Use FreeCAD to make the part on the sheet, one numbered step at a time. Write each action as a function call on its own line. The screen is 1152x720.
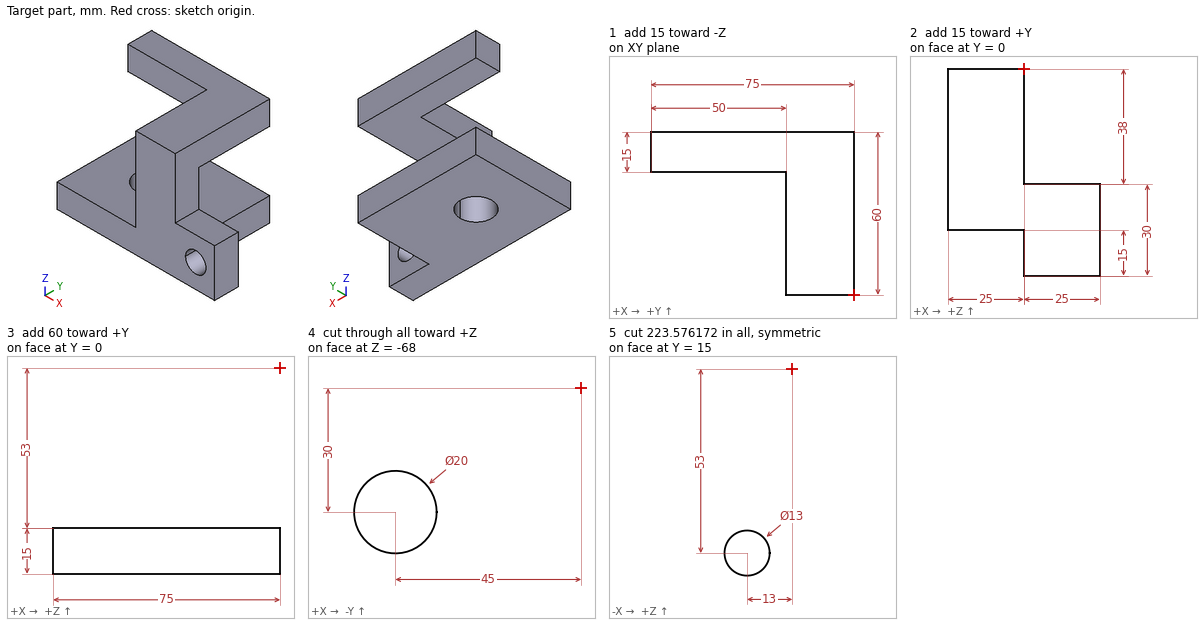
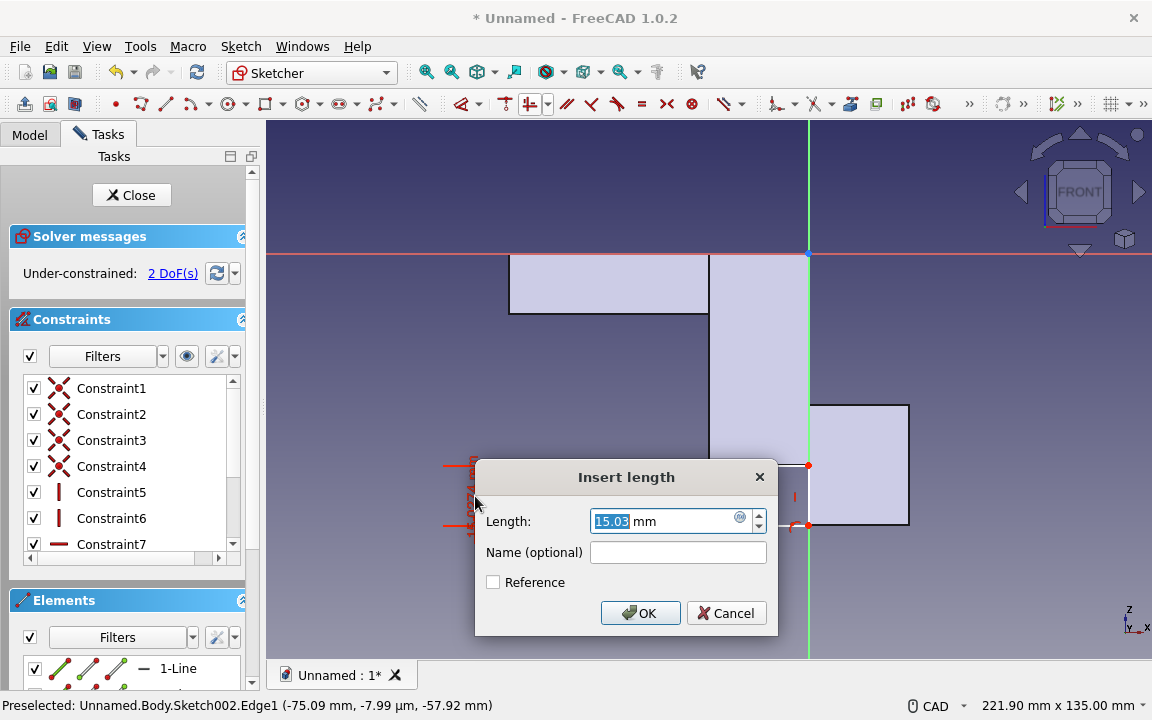
text(15)
key(Return)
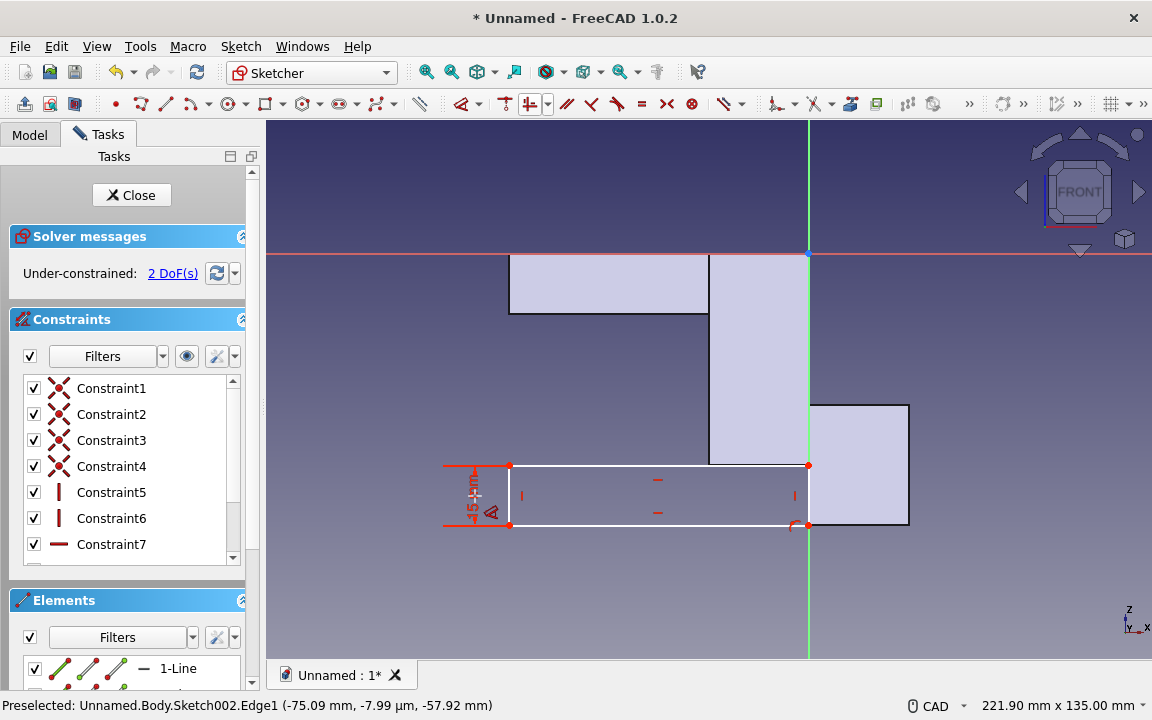
click(599, 526)
click(659, 560)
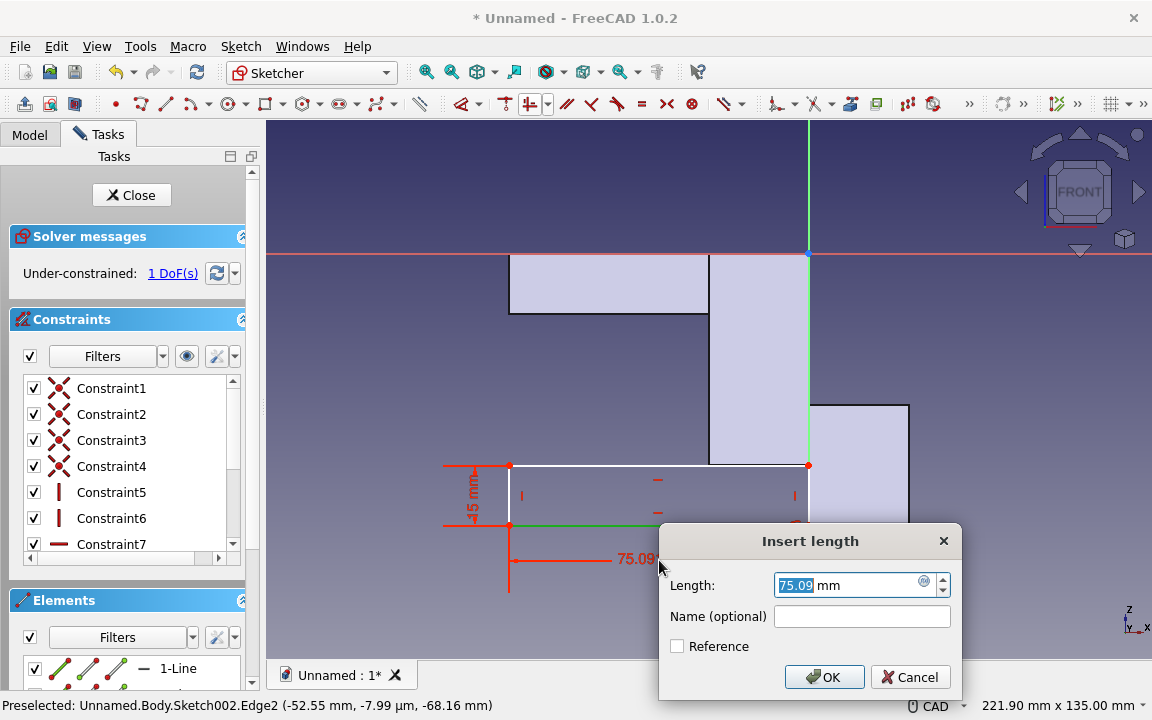
text(75)
key(Return)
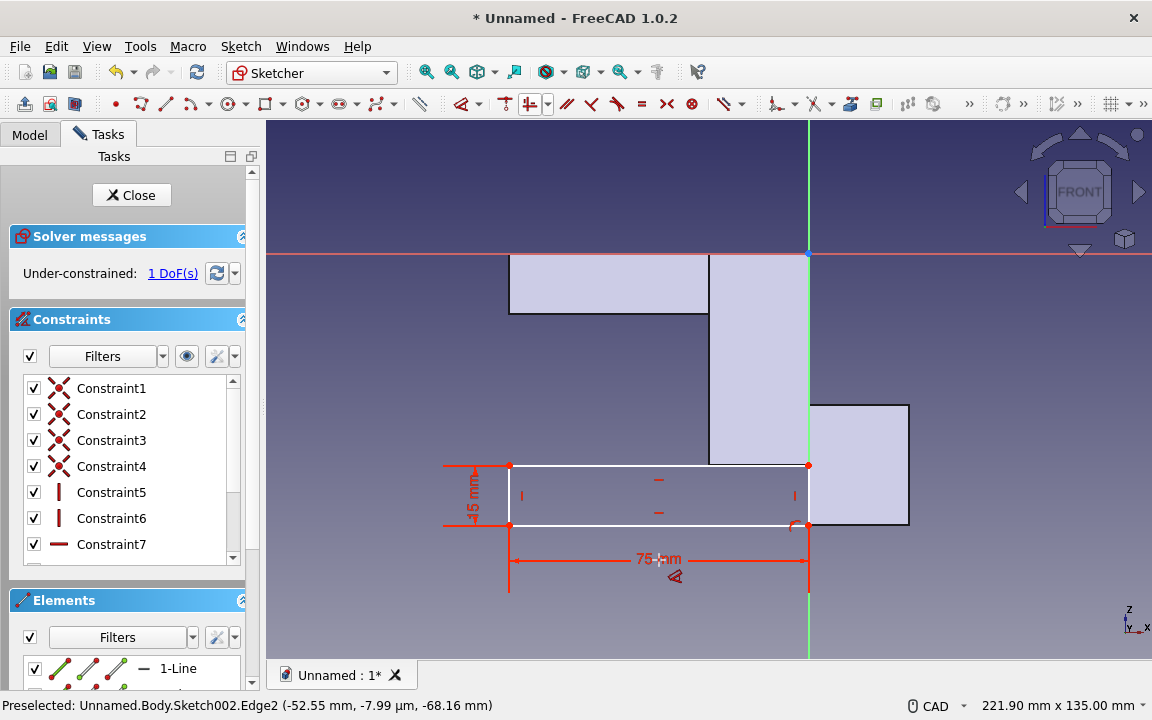
click(509, 466)
click(843, 360)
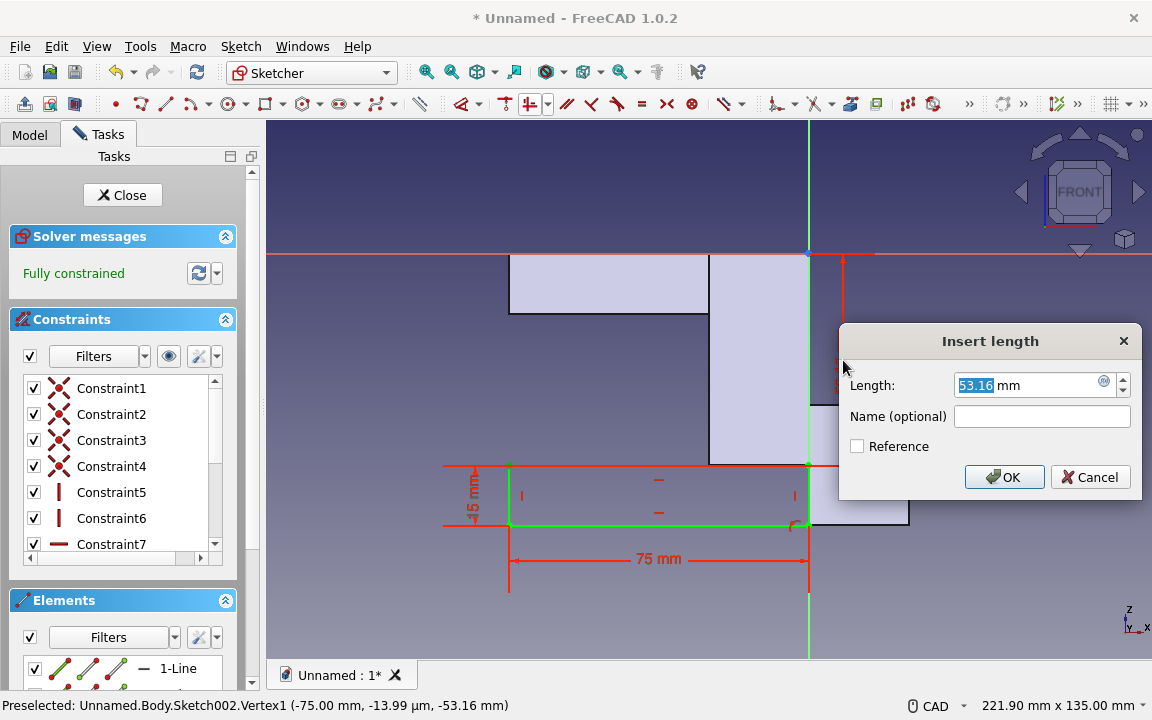
text(53)
key(Return)
key(Escape)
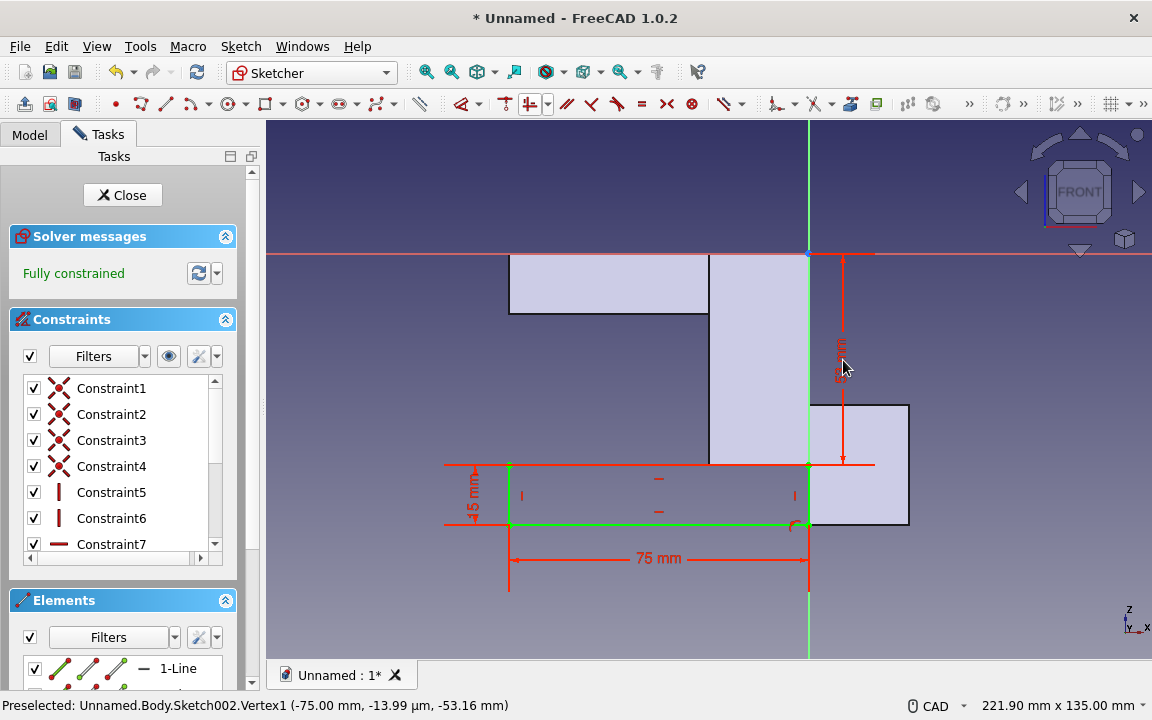
click(123, 195)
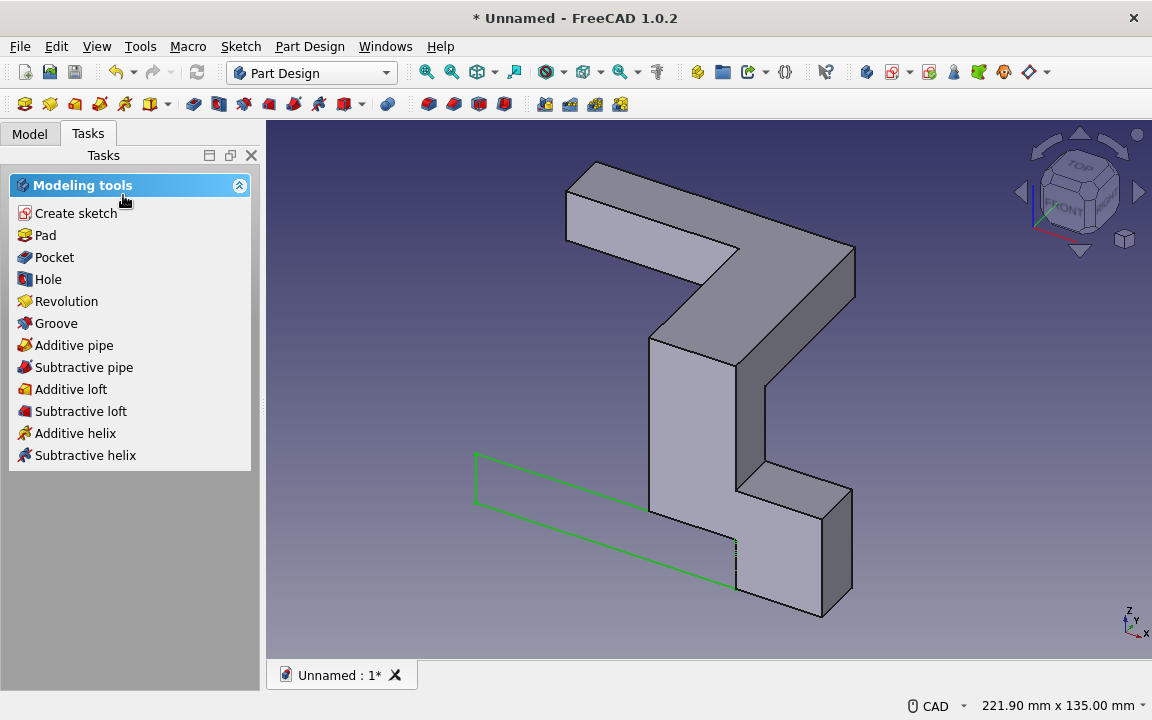
click(25, 104)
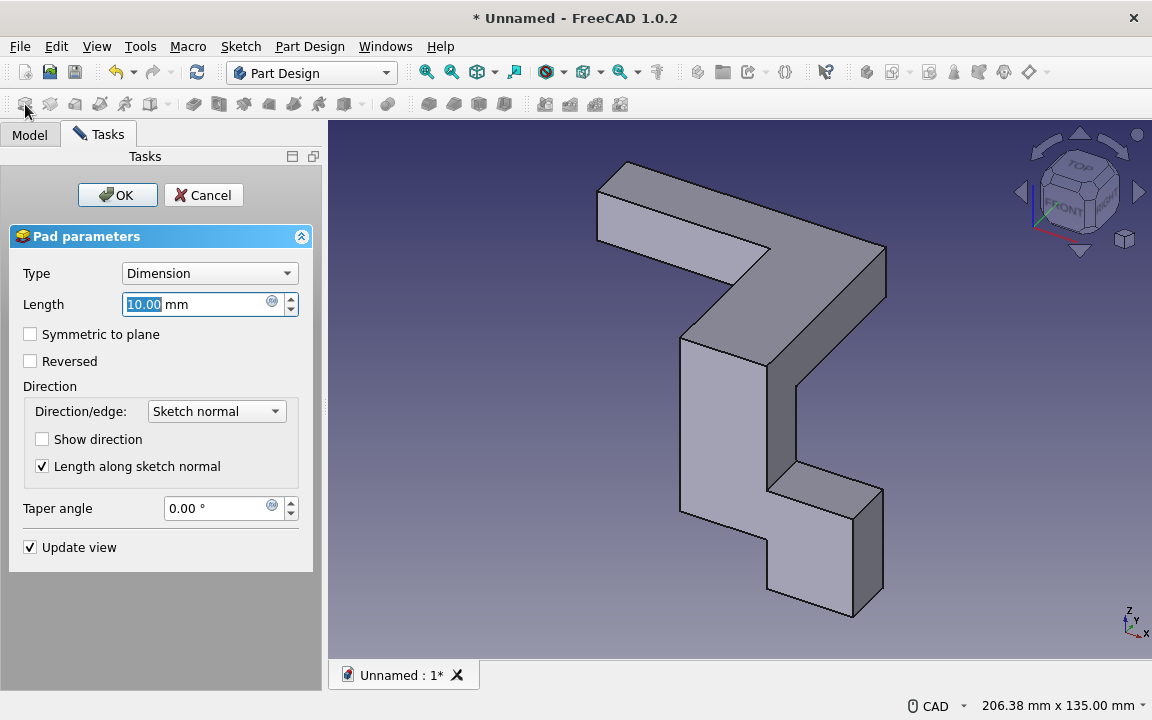
text(60)
key(Tab)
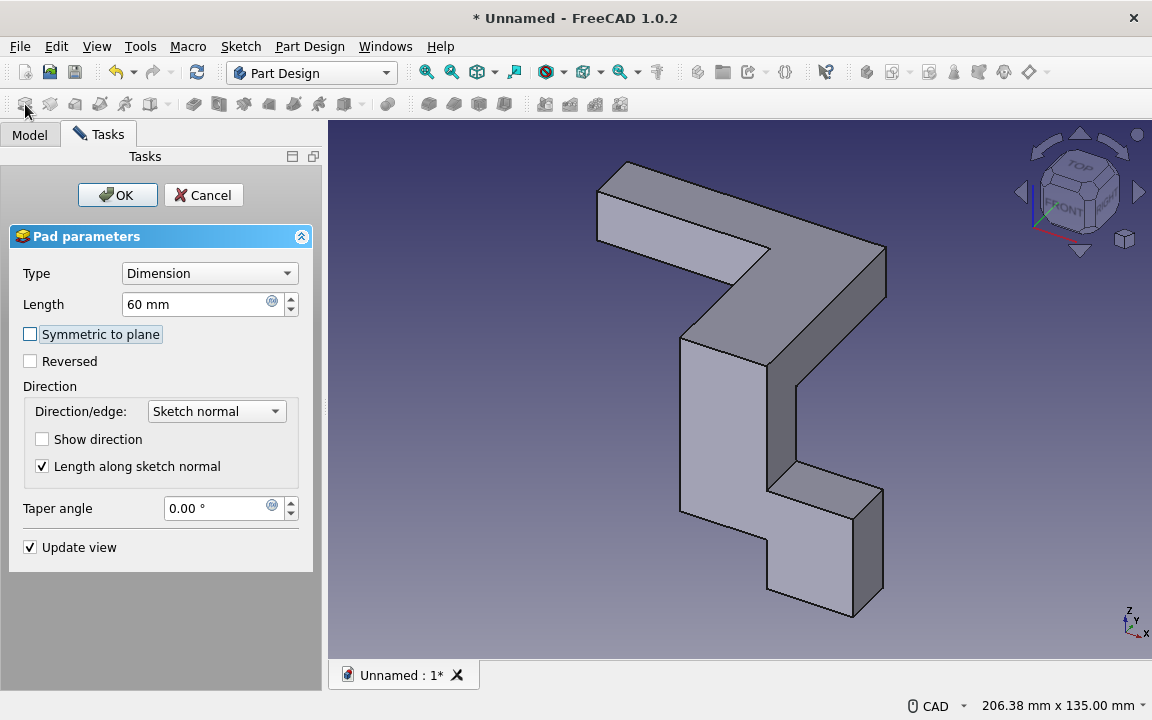
click(31, 361)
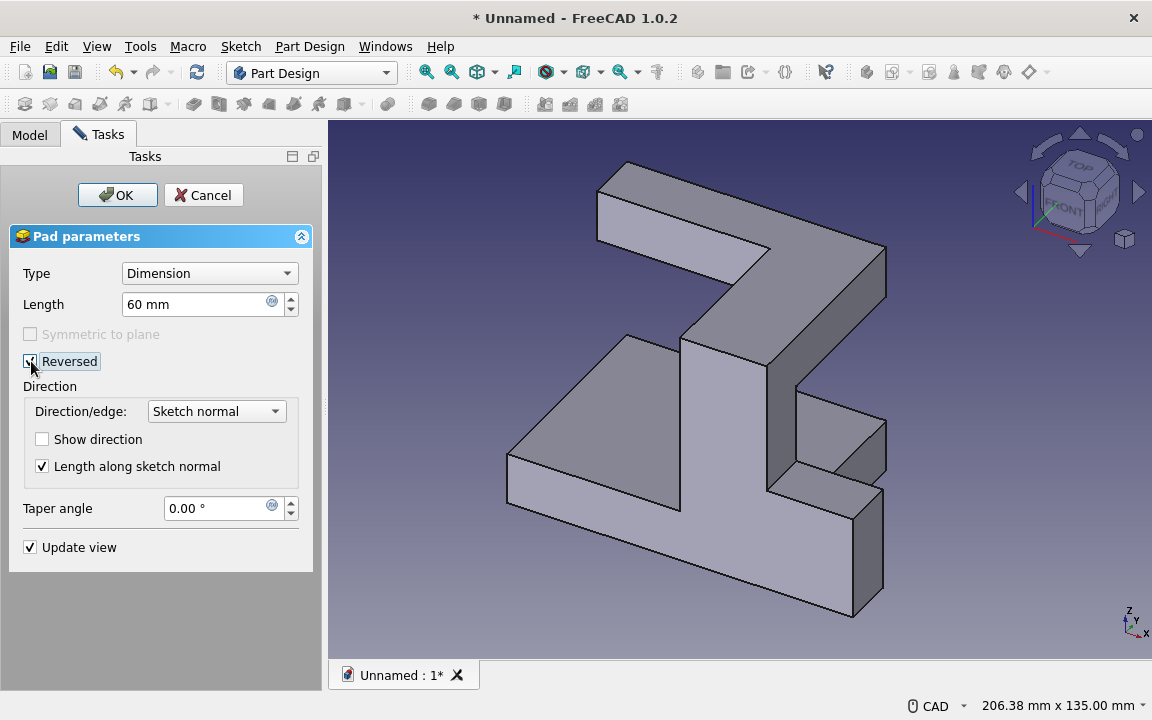
click(118, 195)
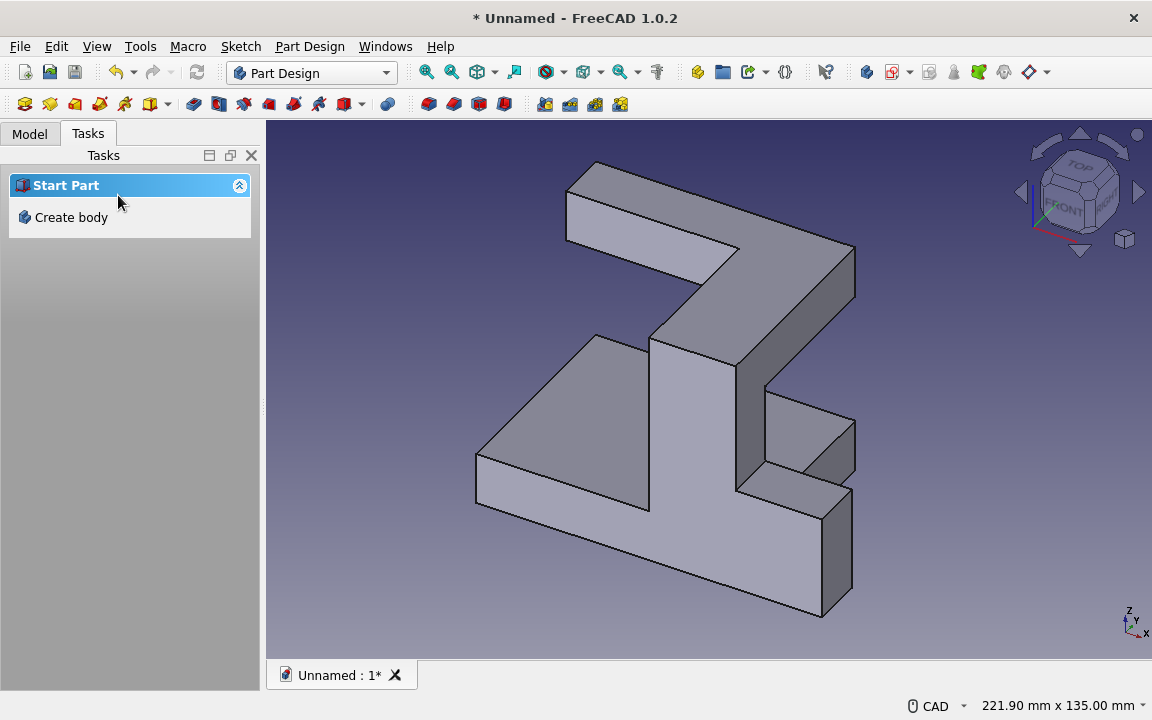
key(5)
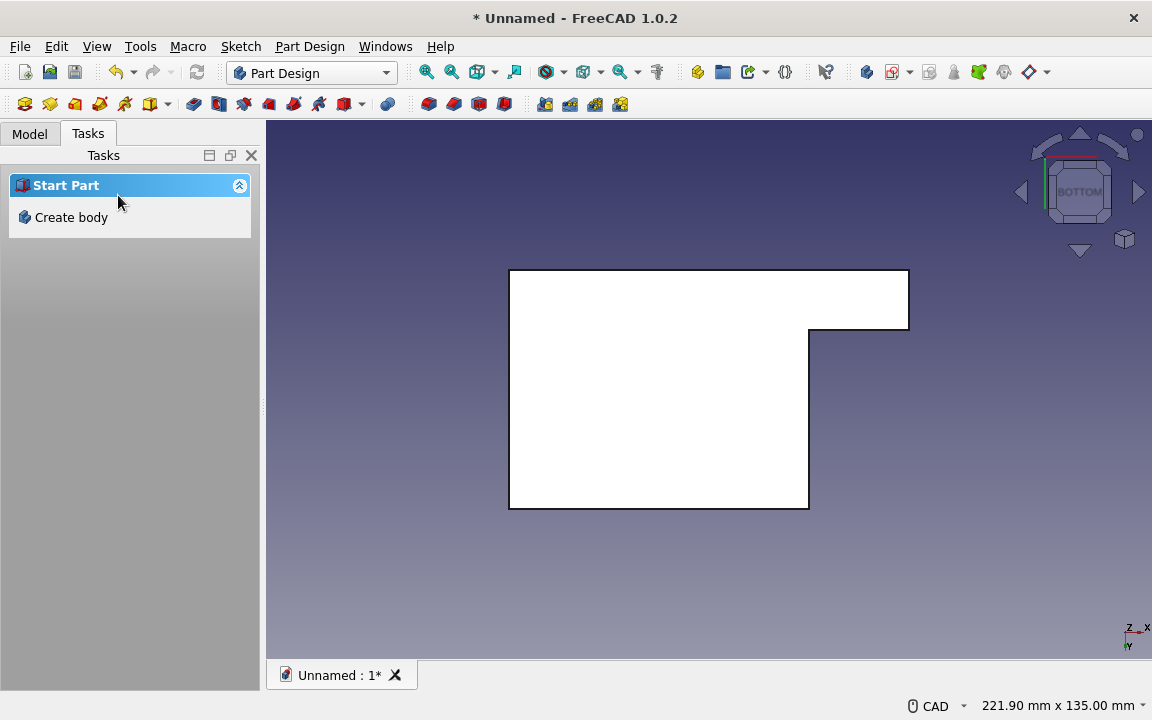
click(652, 388)